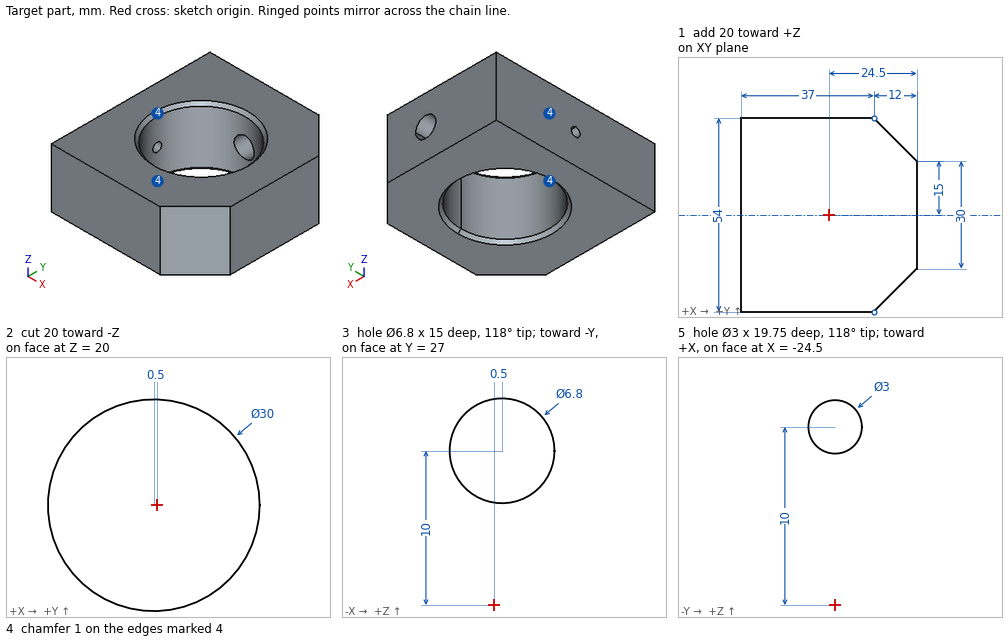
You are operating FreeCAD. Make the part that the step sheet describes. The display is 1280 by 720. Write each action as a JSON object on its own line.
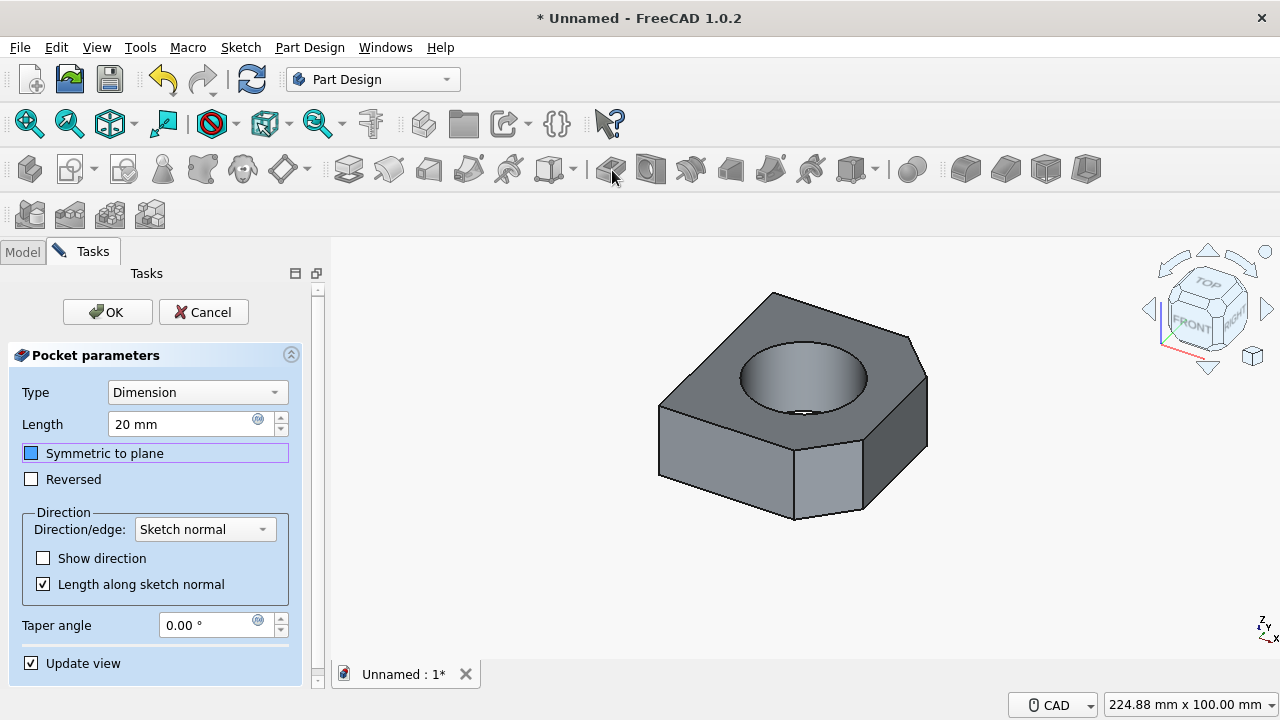
{"action": "left_click", "coordinate": [108, 312]}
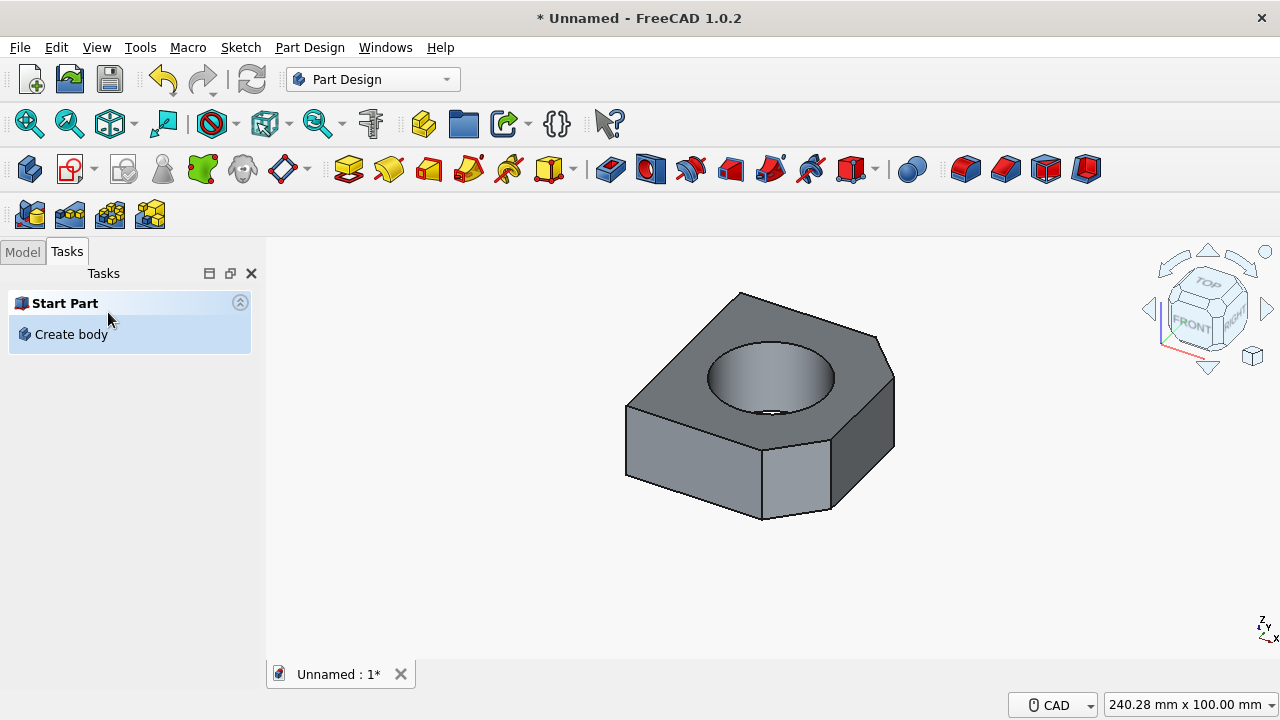
{"action": "key", "text": "4"}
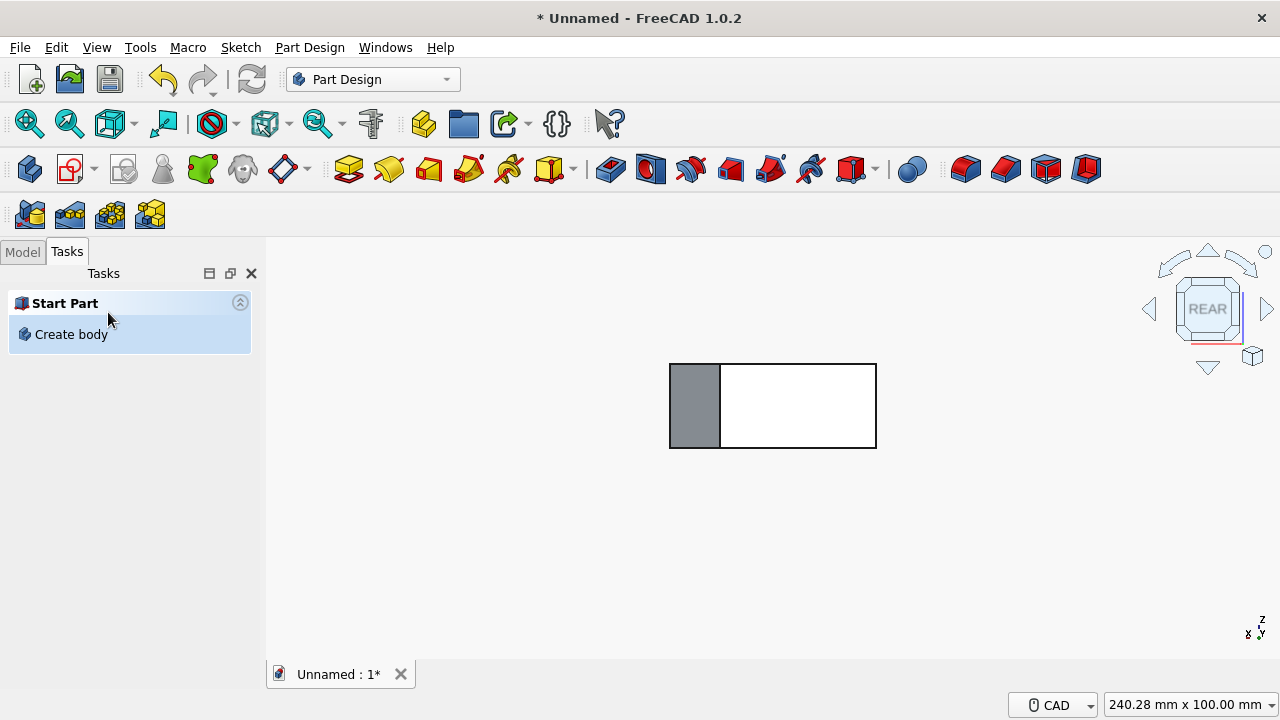
{"action": "key", "text": "v f"}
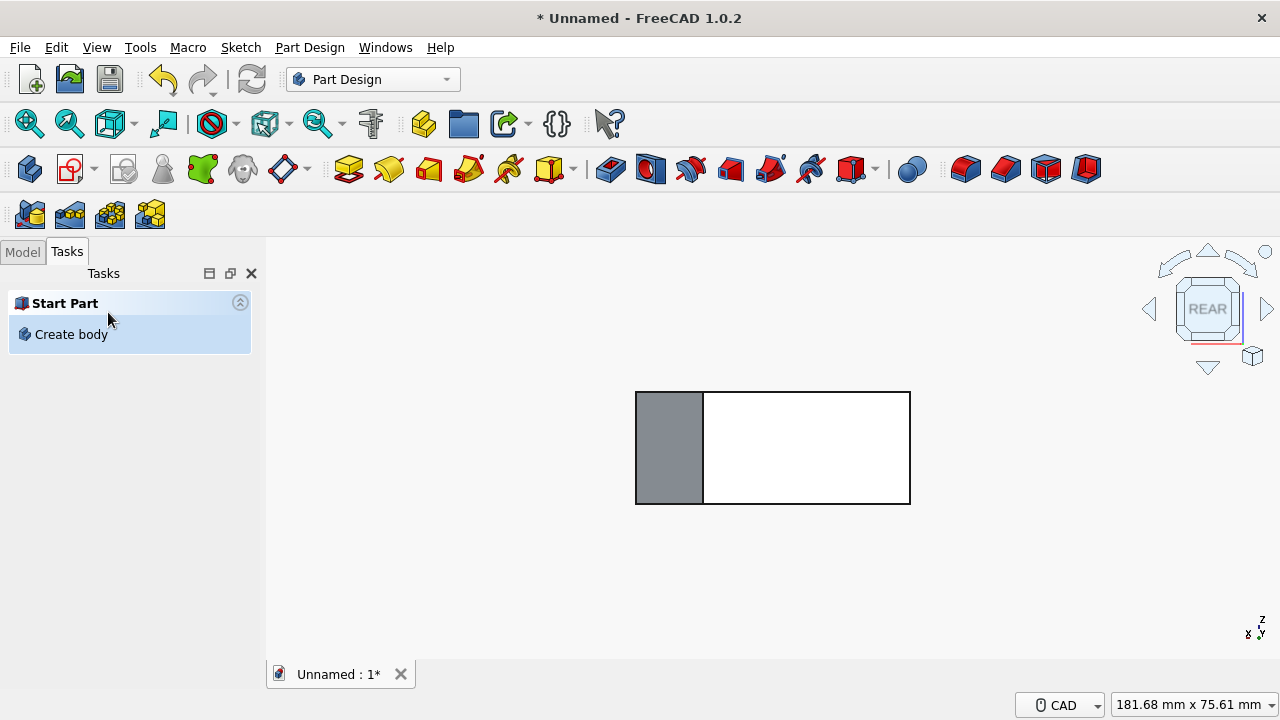
{"action": "left_click", "coordinate": [777, 447]}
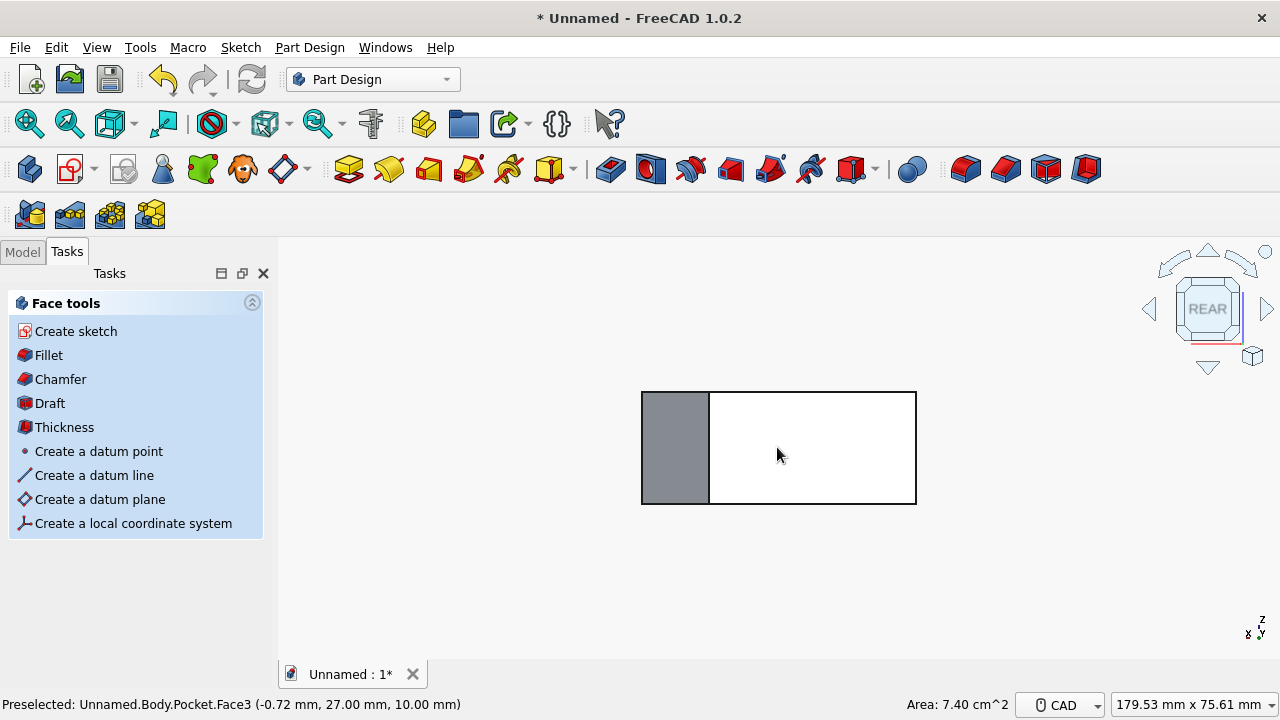
{"action": "left_click", "coordinate": [70, 170]}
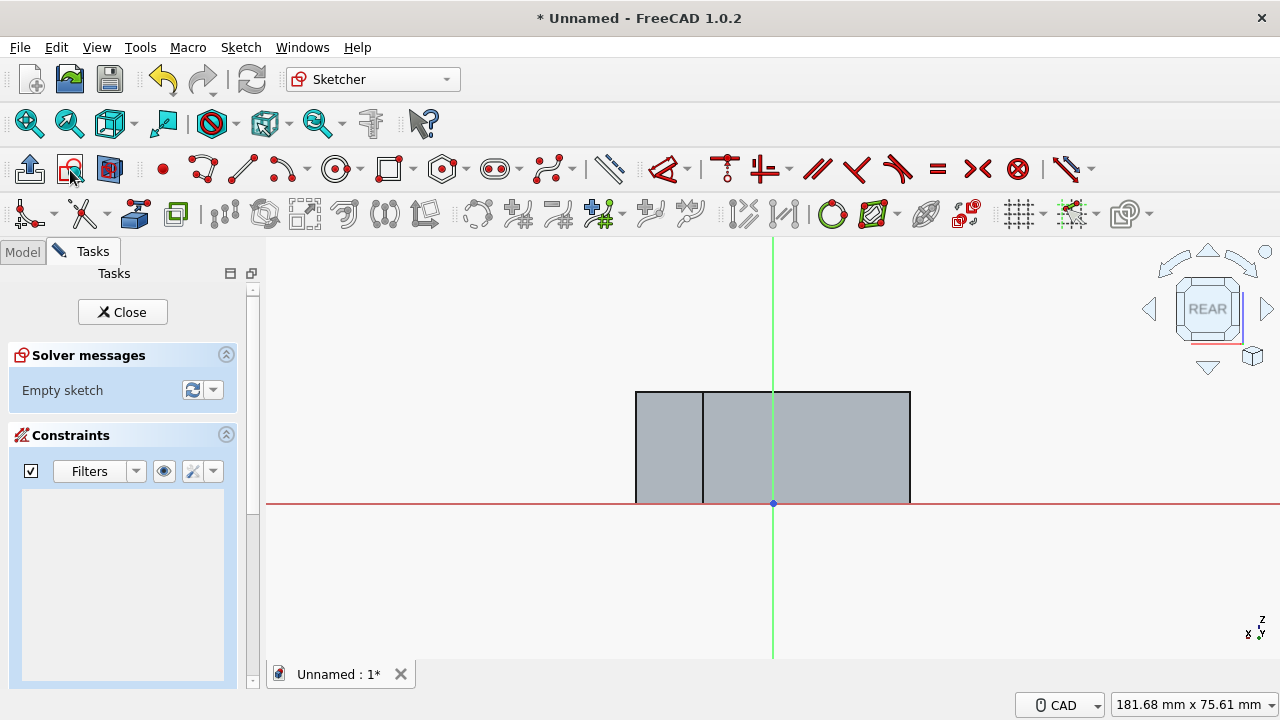
{"action": "scroll", "coordinate": [807, 474], "scroll_direction": "up", "scroll_amount": 6}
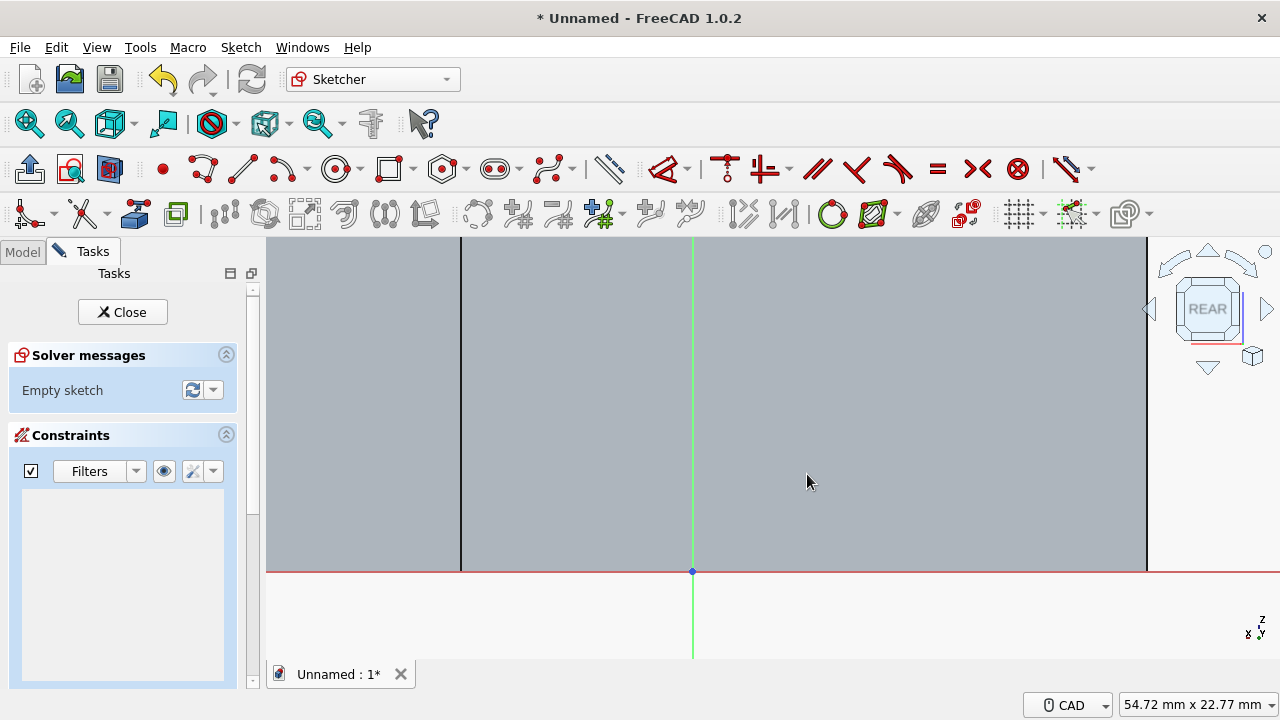
{"action": "key", "text": "g c"}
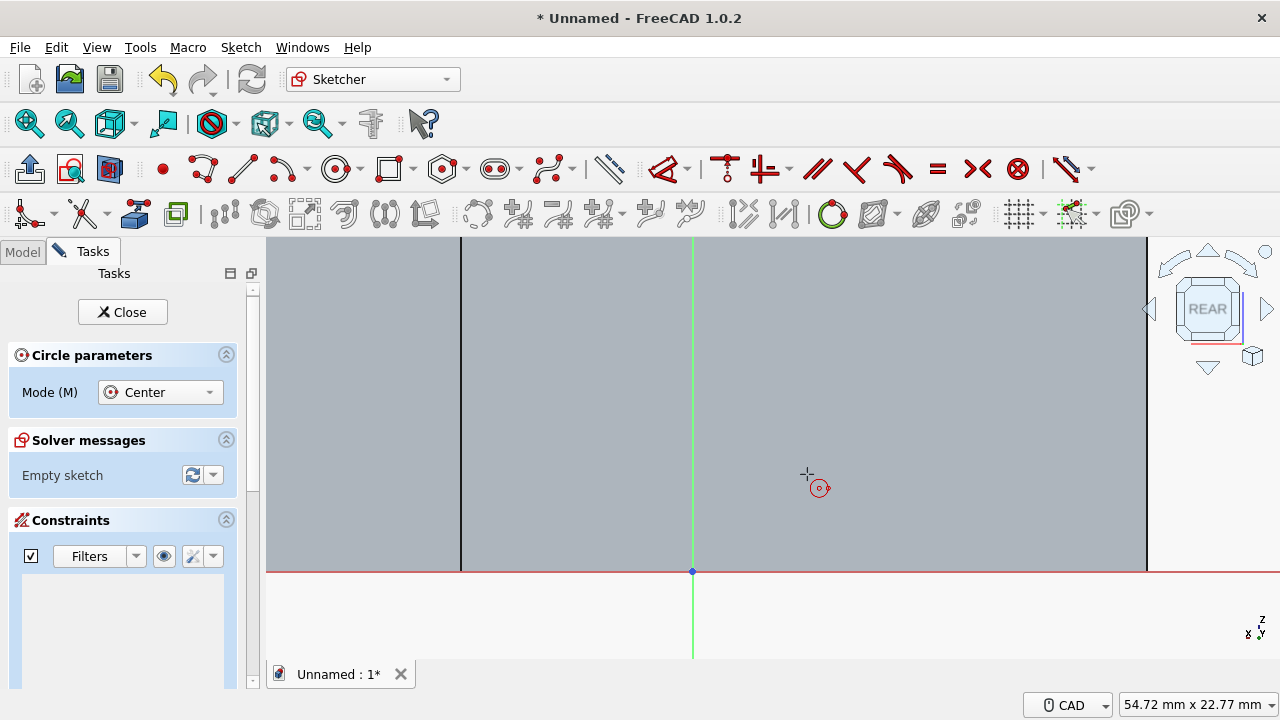
{"action": "scroll", "coordinate": [702, 386], "scroll_direction": "up", "scroll_amount": 3}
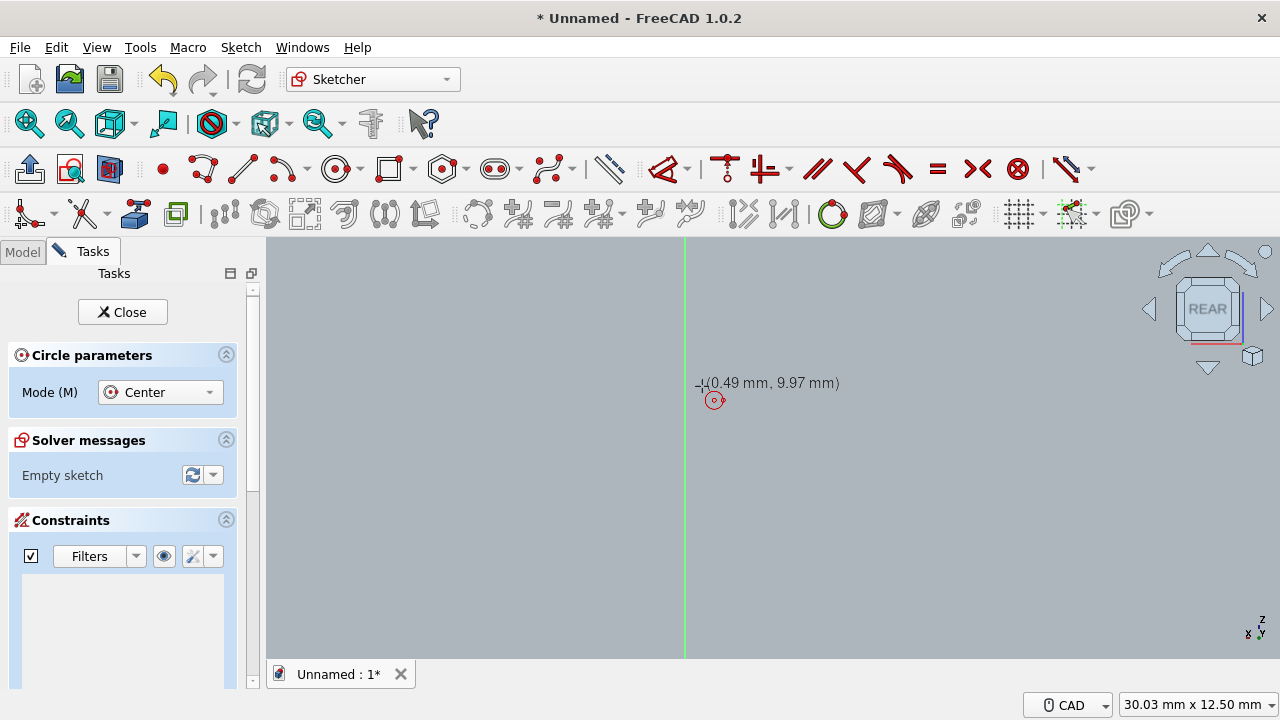
{"action": "left_click", "coordinate": [702, 386]}
{"action": "left_click", "coordinate": [783, 305]}
{"action": "key", "text": "Escape"}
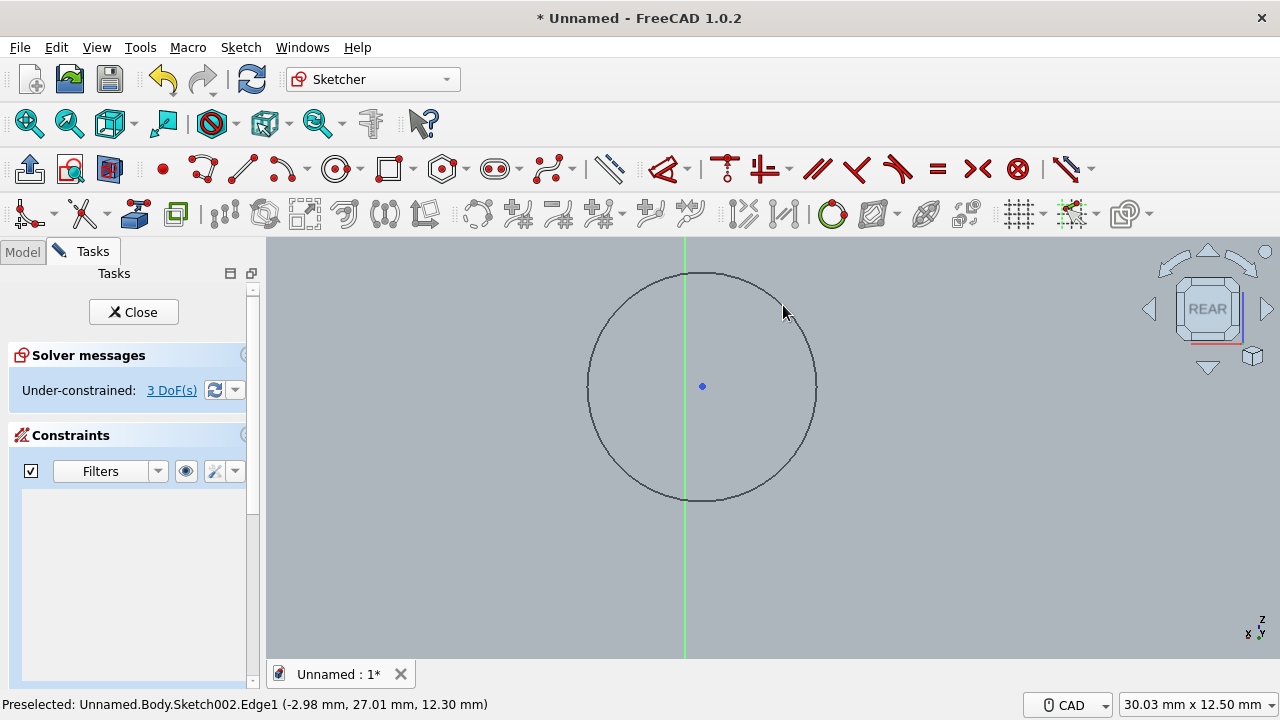
{"action": "key", "text": "d"}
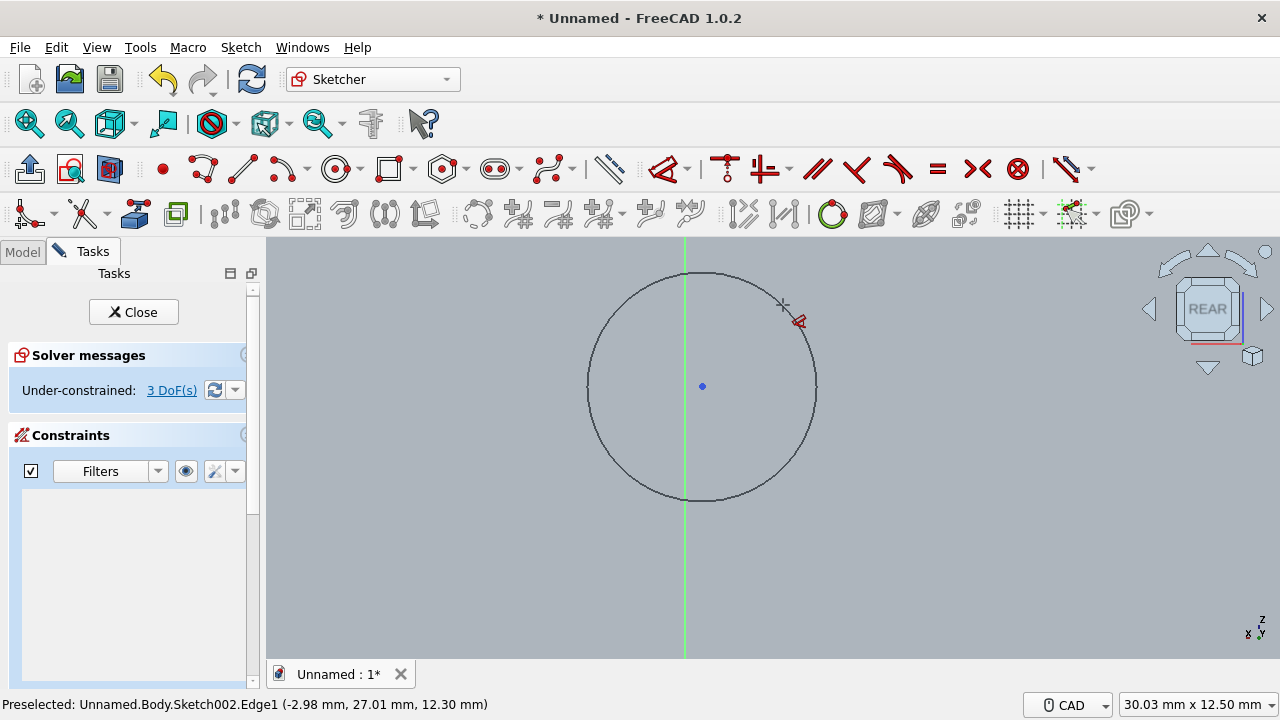
{"action": "left_click", "coordinate": [783, 306]}
{"action": "left_click", "coordinate": [806, 283]}